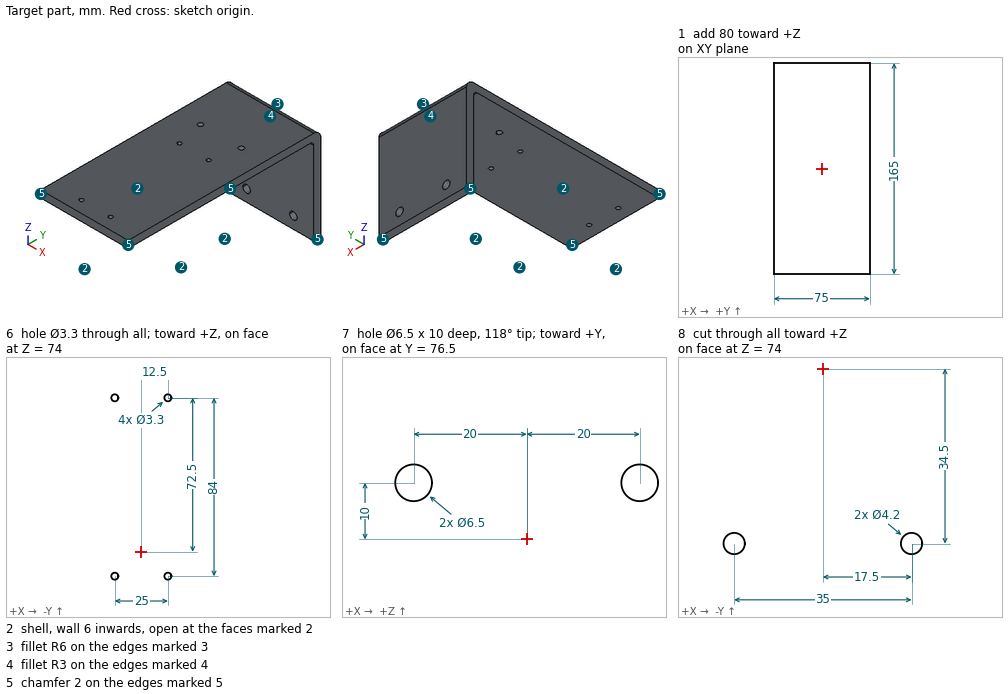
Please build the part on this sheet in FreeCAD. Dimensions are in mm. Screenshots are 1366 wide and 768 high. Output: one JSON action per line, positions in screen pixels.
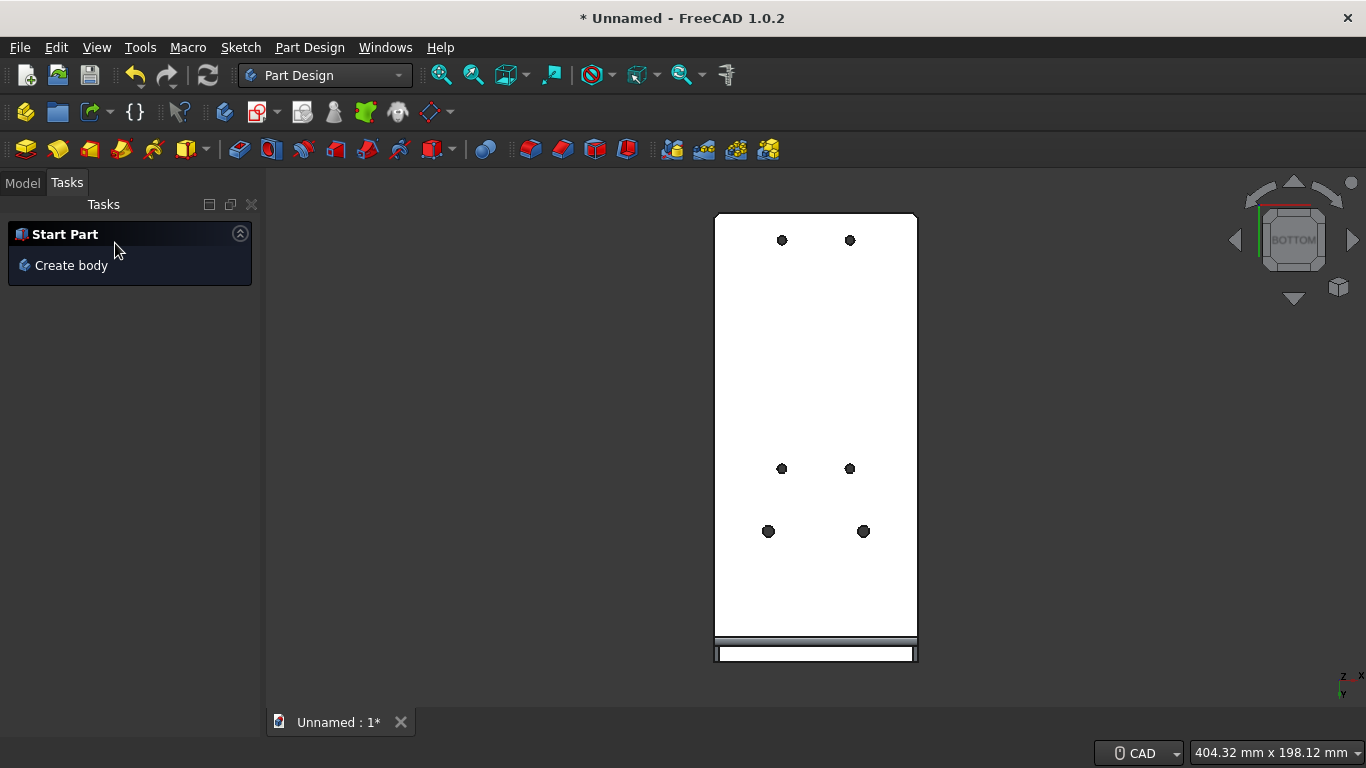
{"action": "key", "text": "0"}